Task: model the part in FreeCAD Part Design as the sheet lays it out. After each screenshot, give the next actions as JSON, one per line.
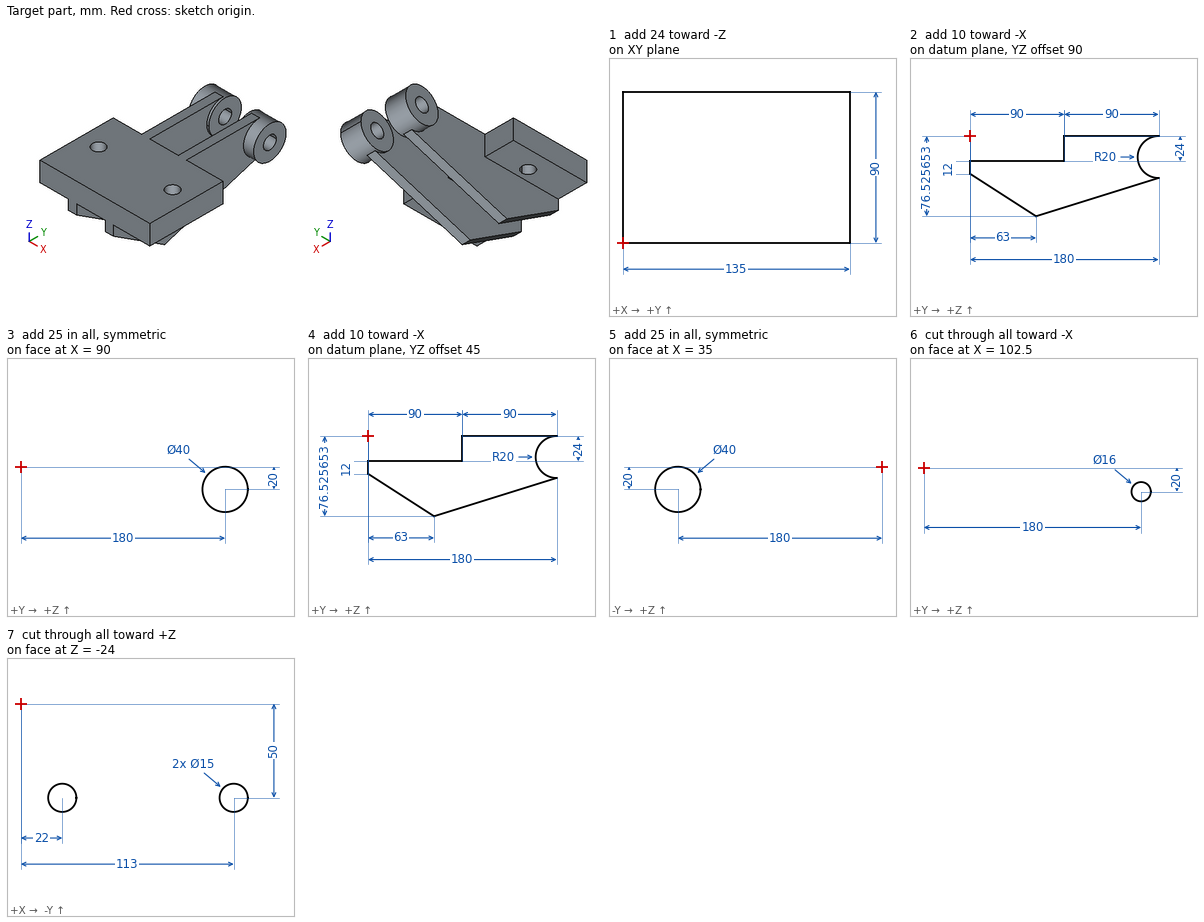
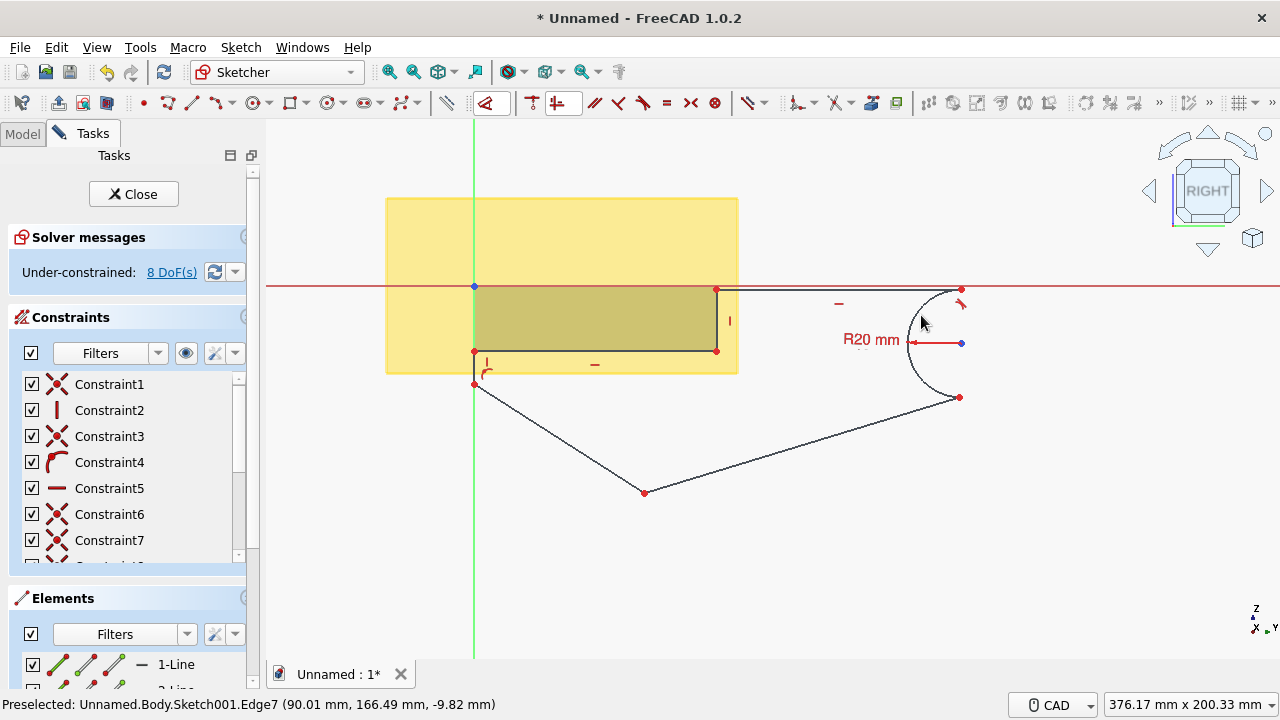
{"action": "left_click", "coordinate": [962, 290]}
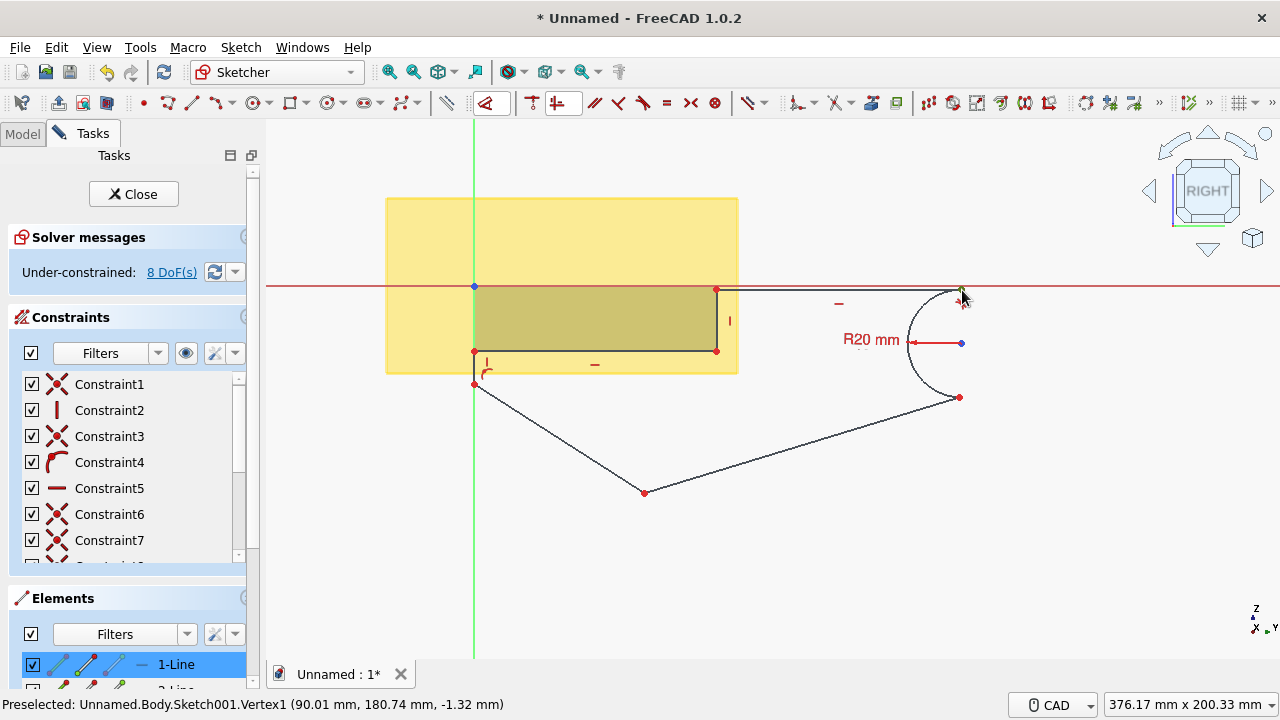
{"action": "left_click", "coordinate": [353, 286]}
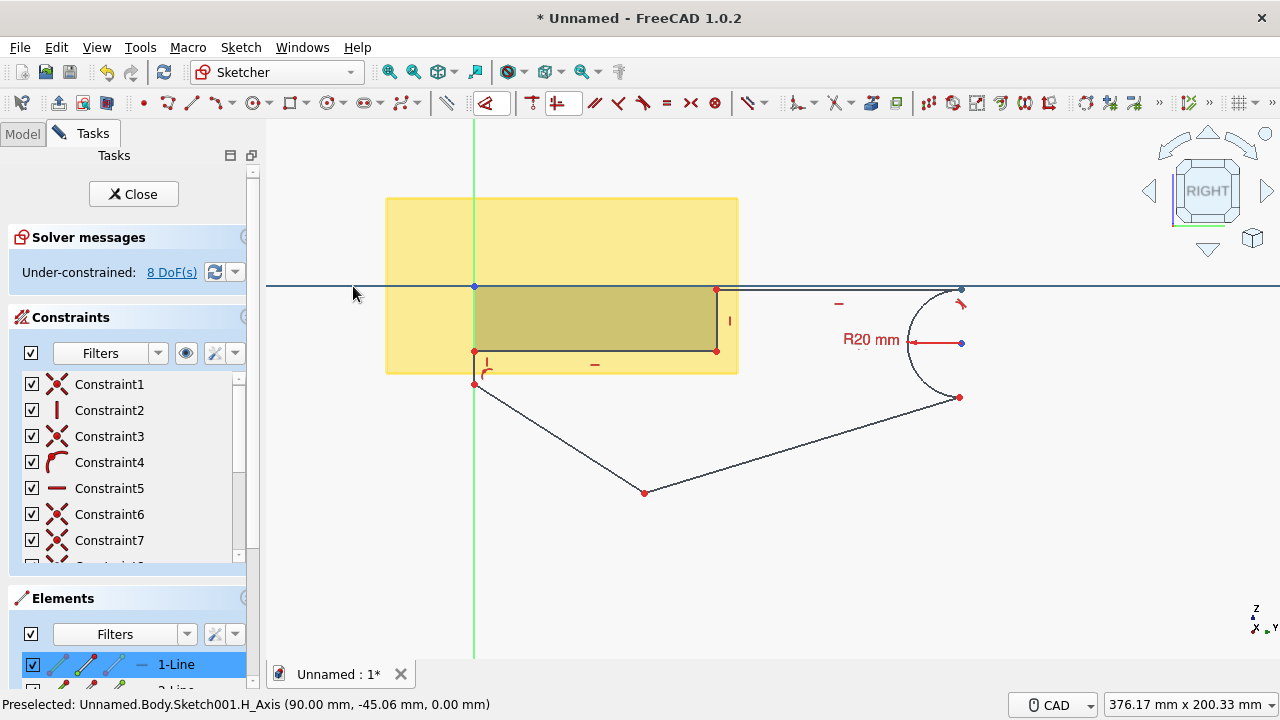
{"action": "left_click", "coordinate": [532, 104]}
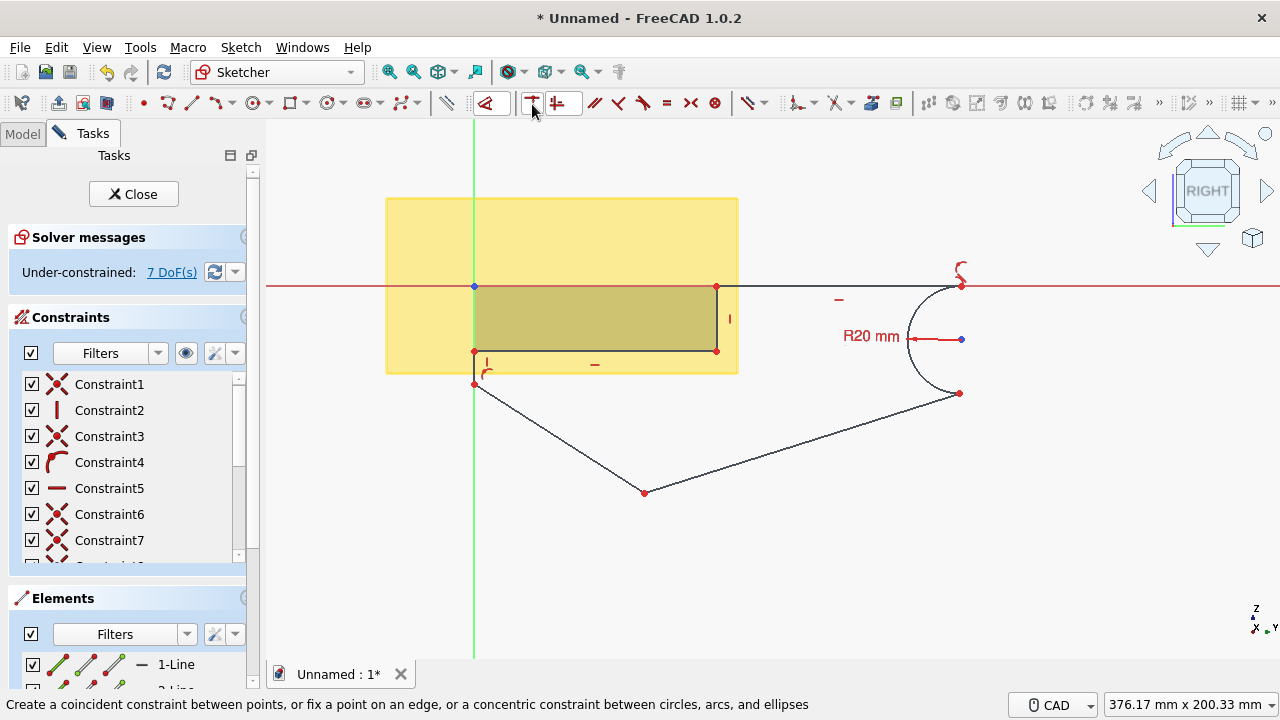
{"action": "left_click", "coordinate": [888, 286]}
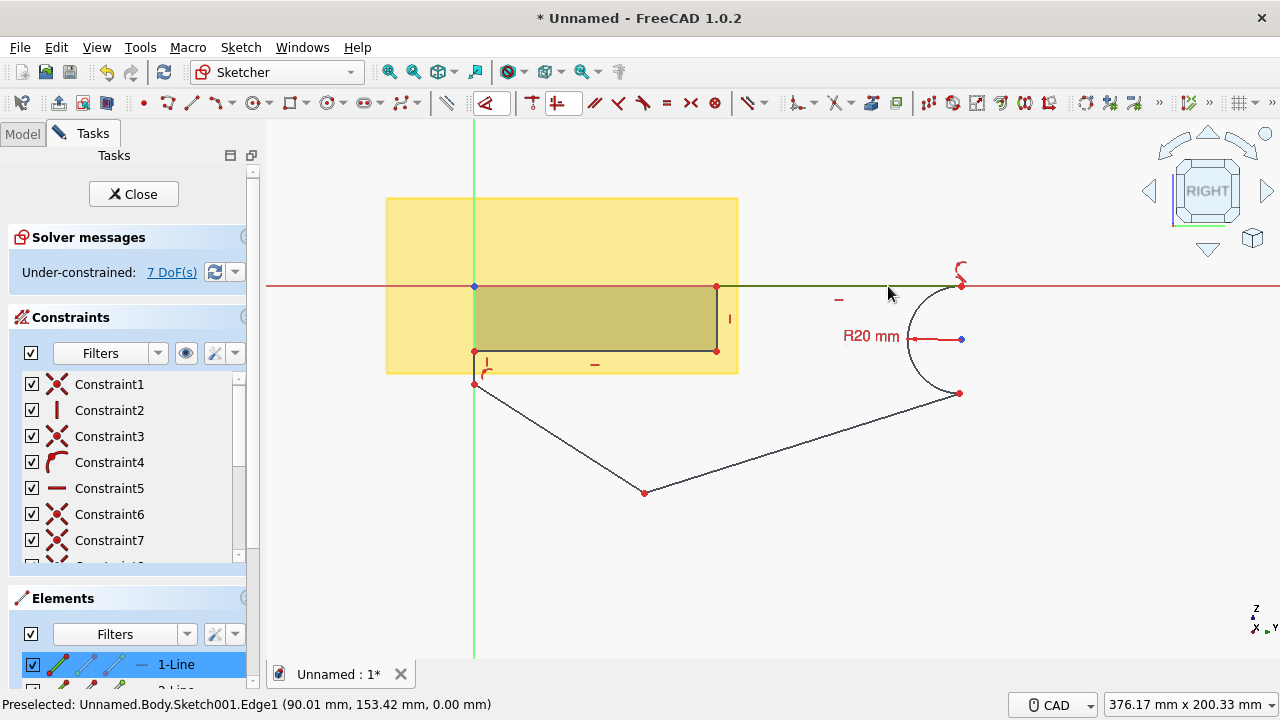
{"action": "key", "text": "l"}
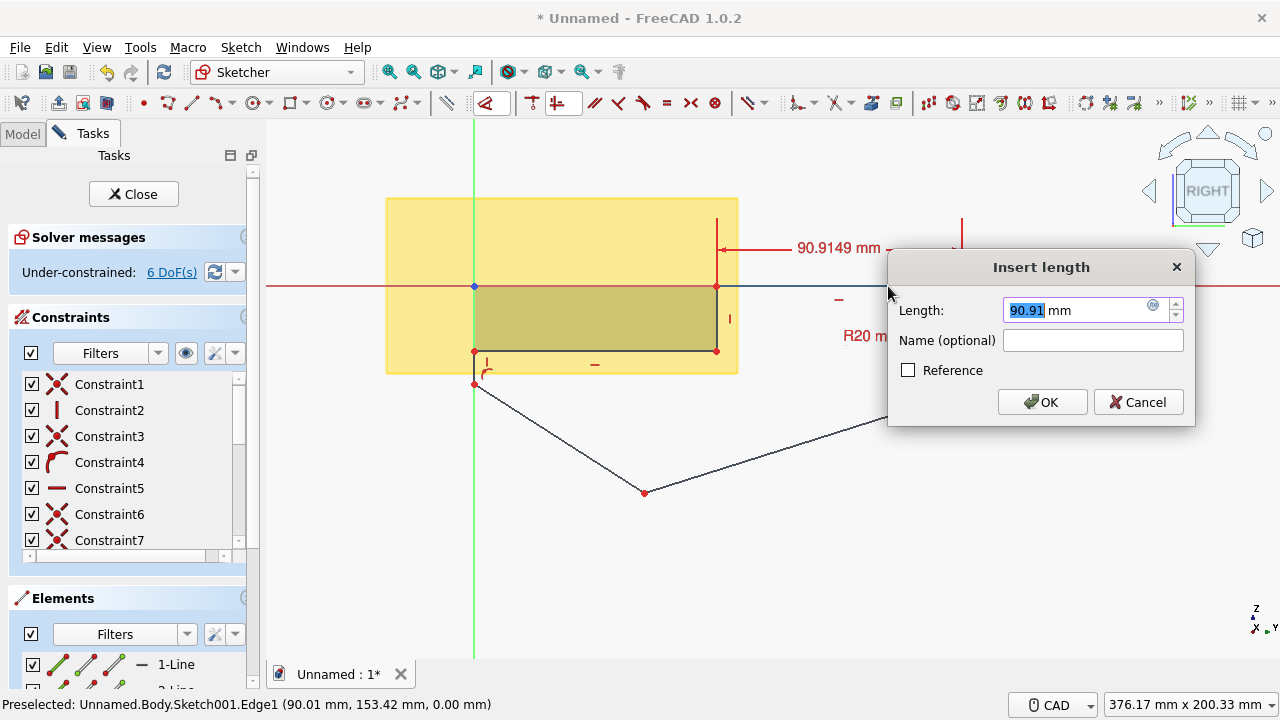
{"action": "type", "text": "90"}
{"action": "key", "text": "Return"}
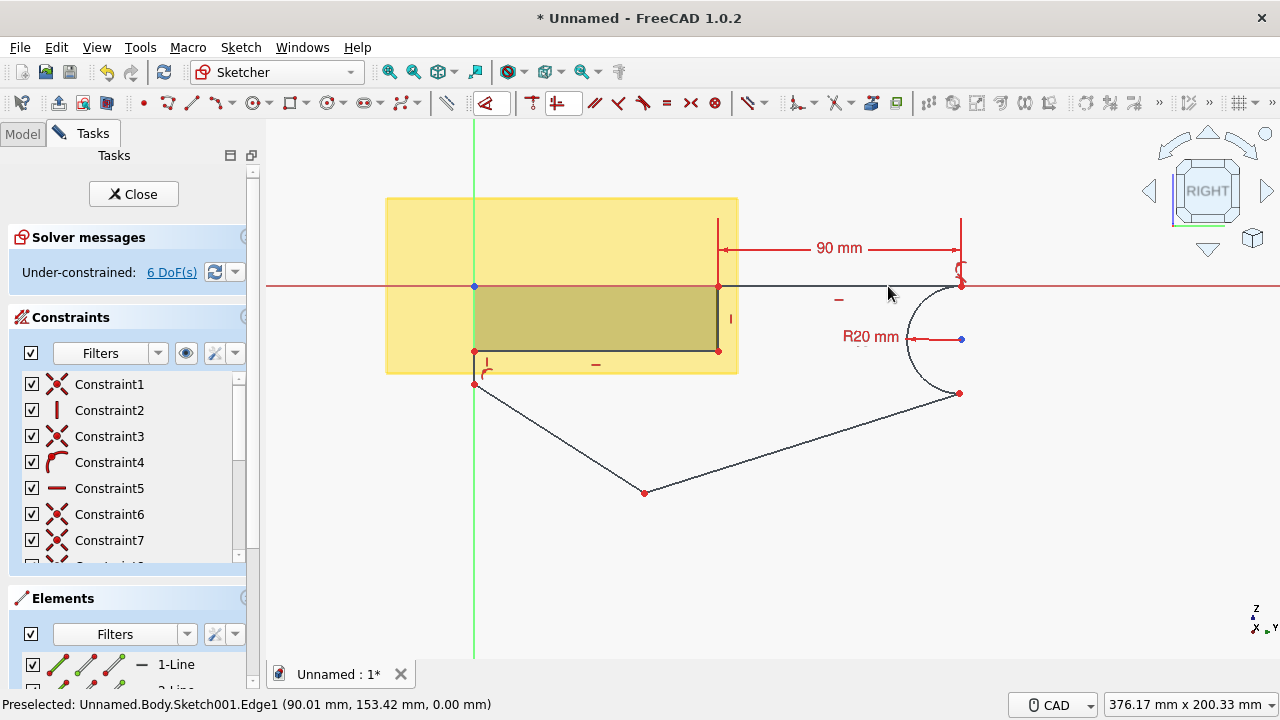
{"action": "left_click", "coordinate": [718, 306]}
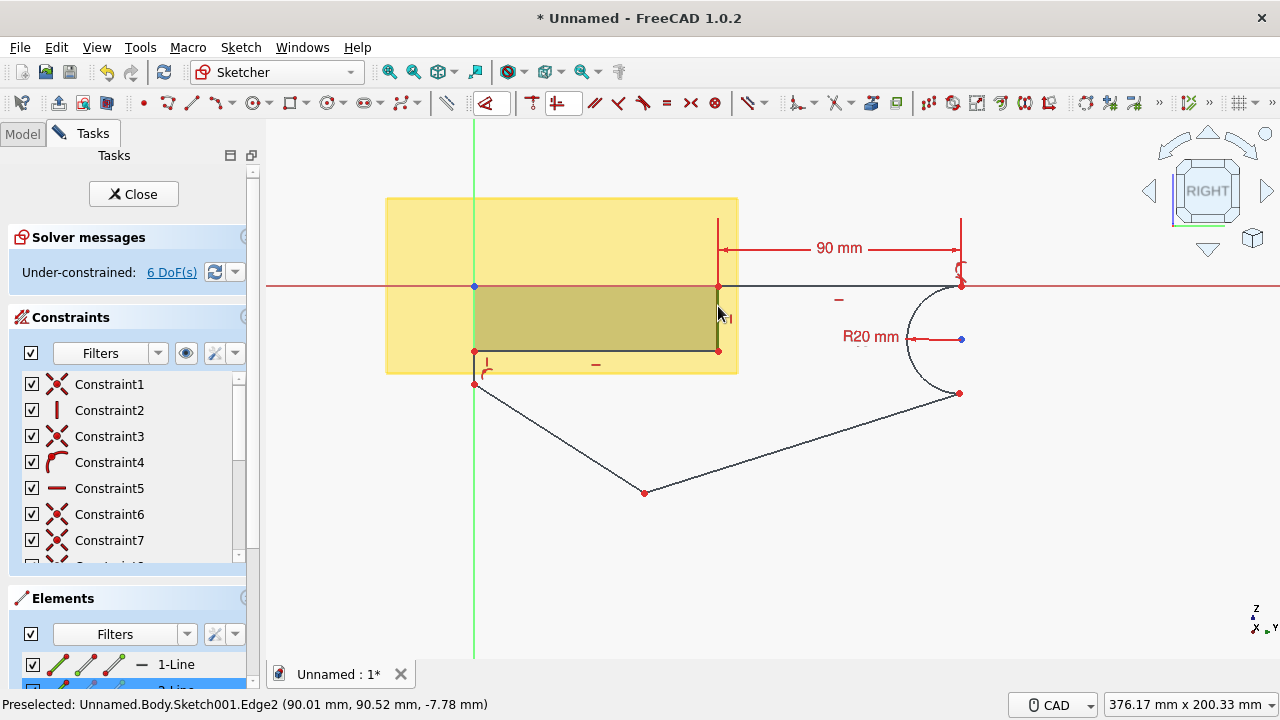
{"action": "key", "text": "i"}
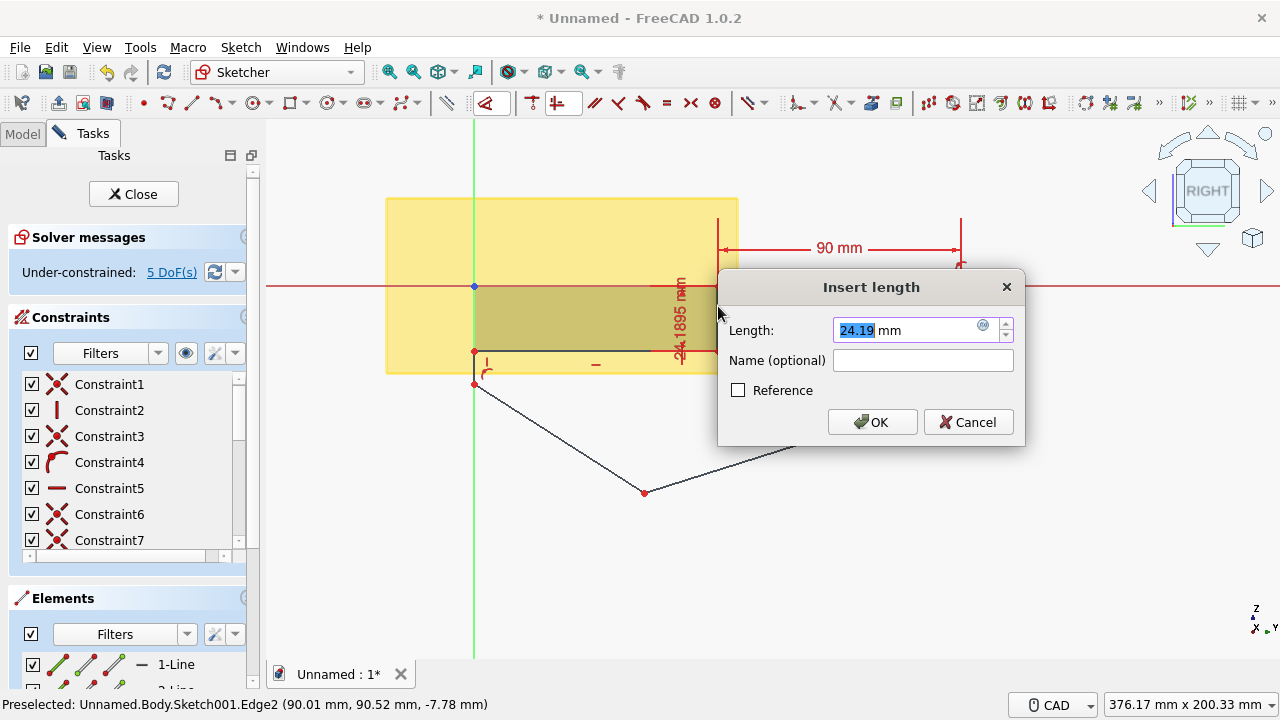
{"action": "type", "text": "24"}
{"action": "key", "text": "Return"}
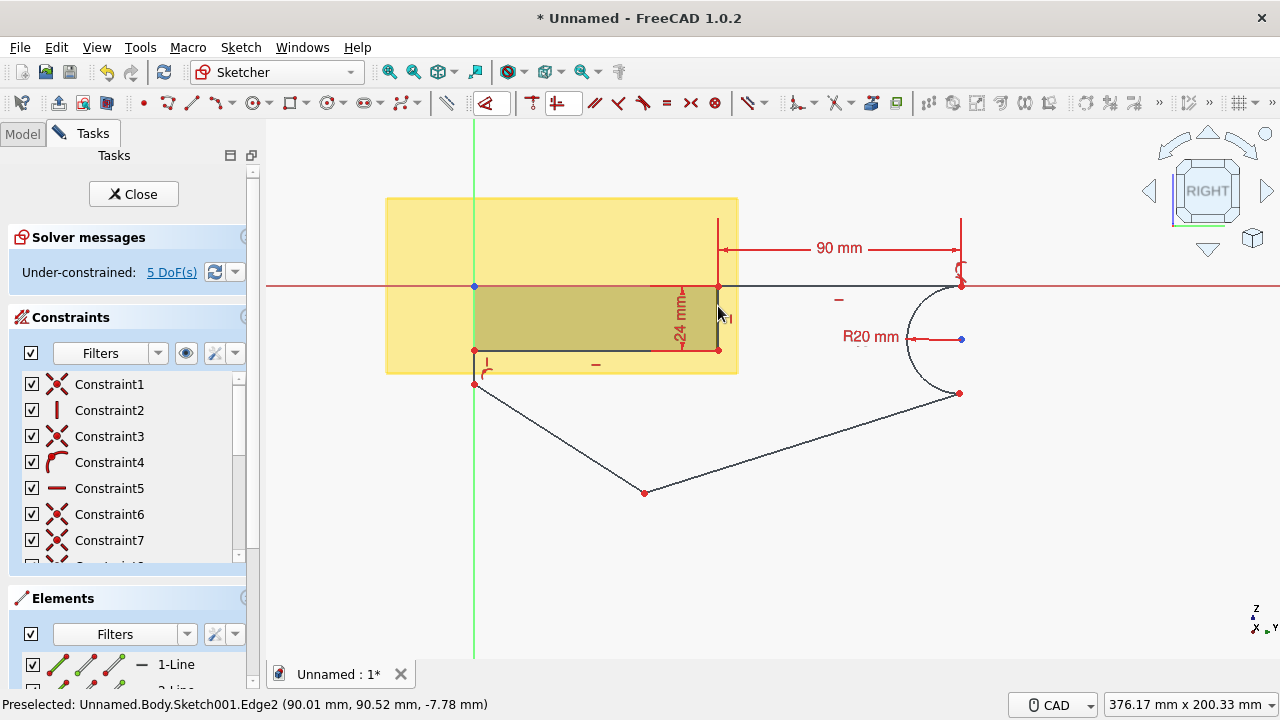
{"action": "left_click", "coordinate": [645, 351]}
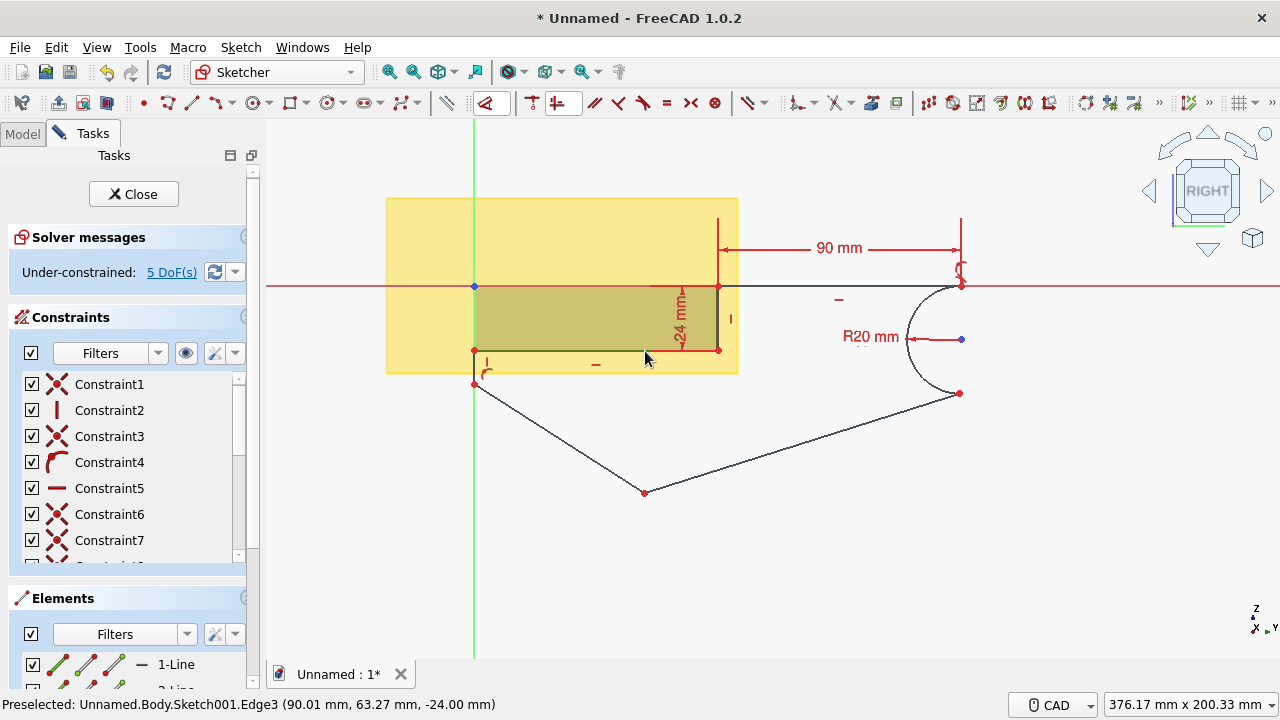
{"action": "key", "text": "l"}